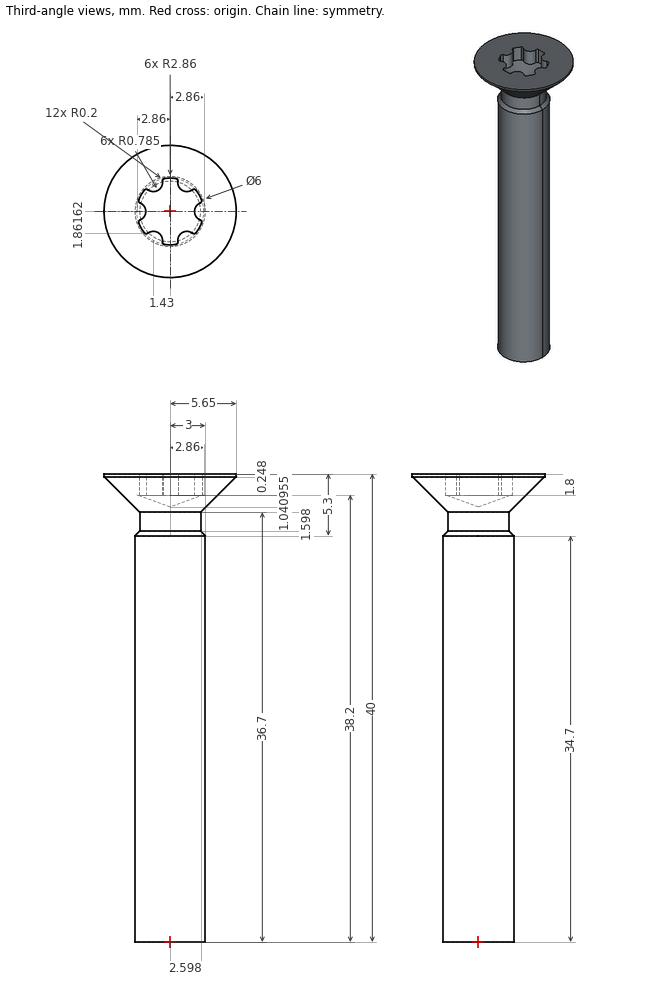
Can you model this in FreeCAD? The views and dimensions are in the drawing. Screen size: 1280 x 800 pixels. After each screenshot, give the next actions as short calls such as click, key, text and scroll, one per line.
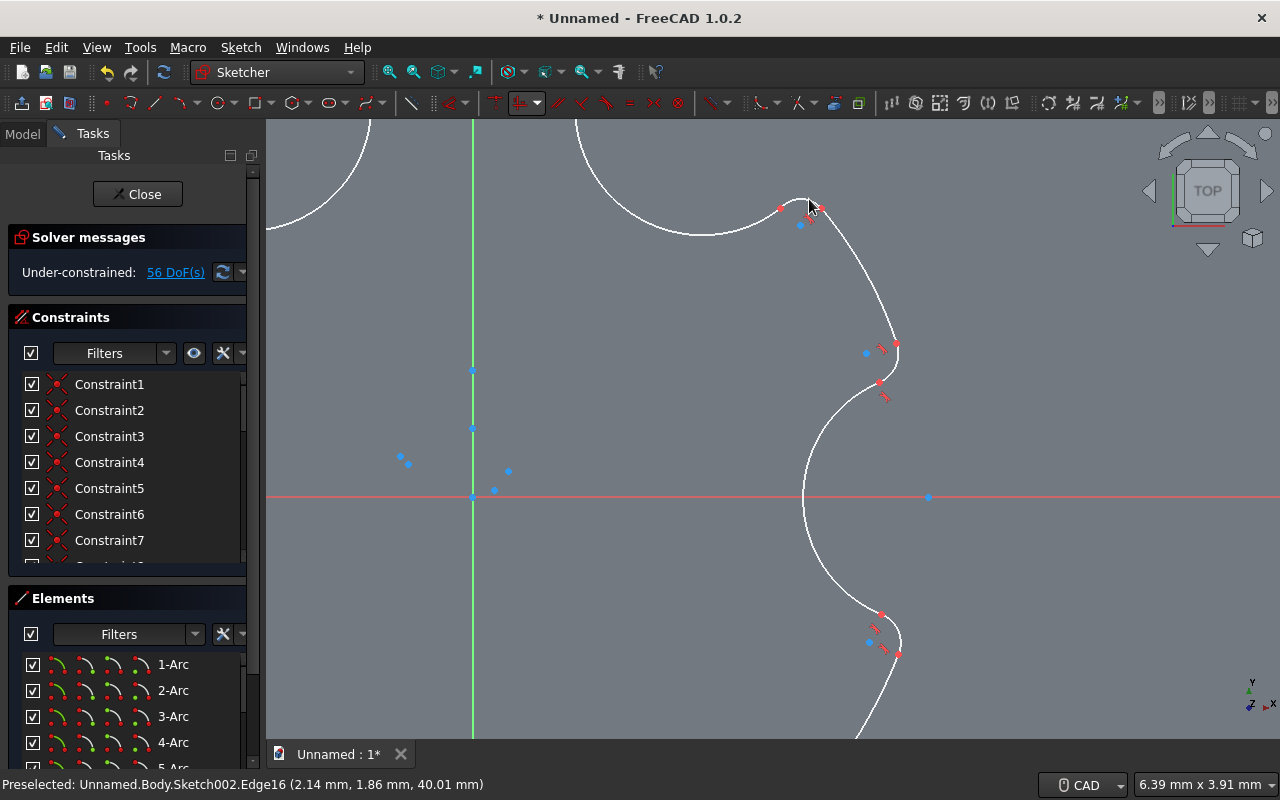
click(810, 201)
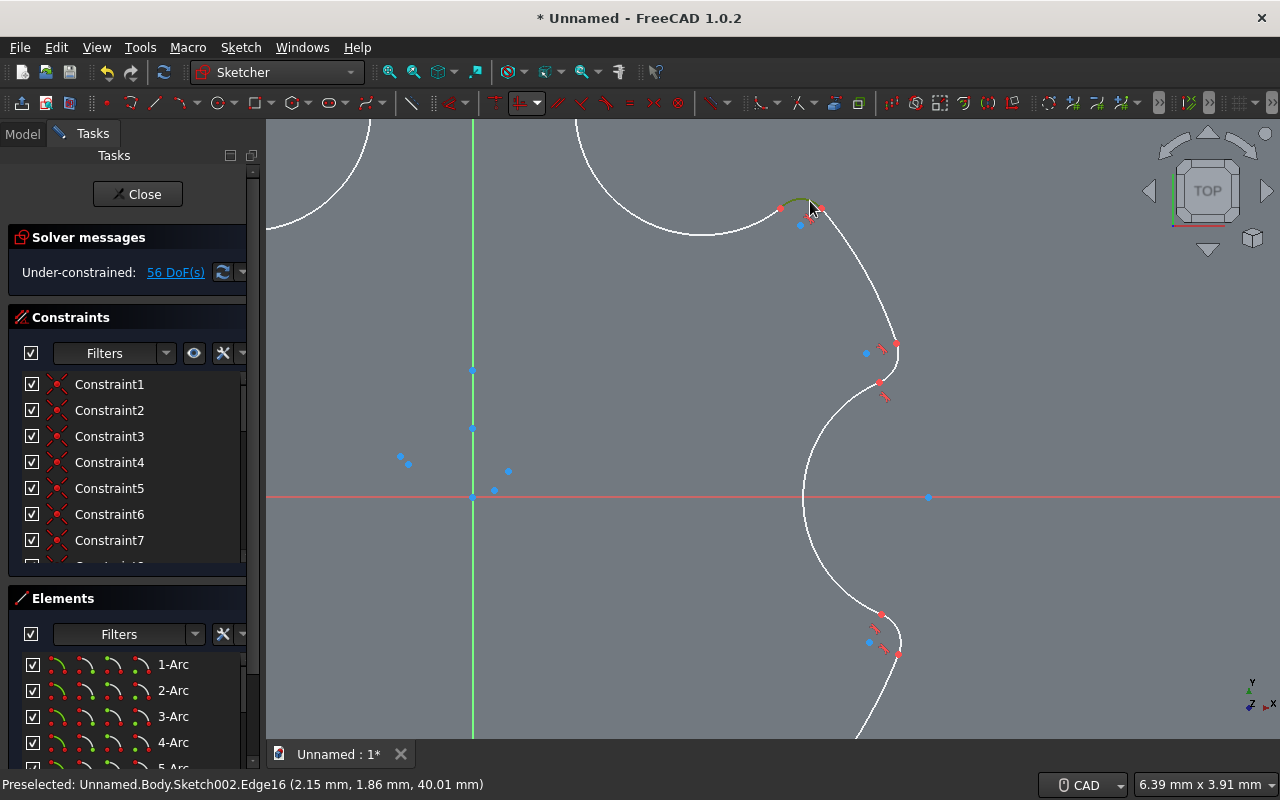
click(594, 175)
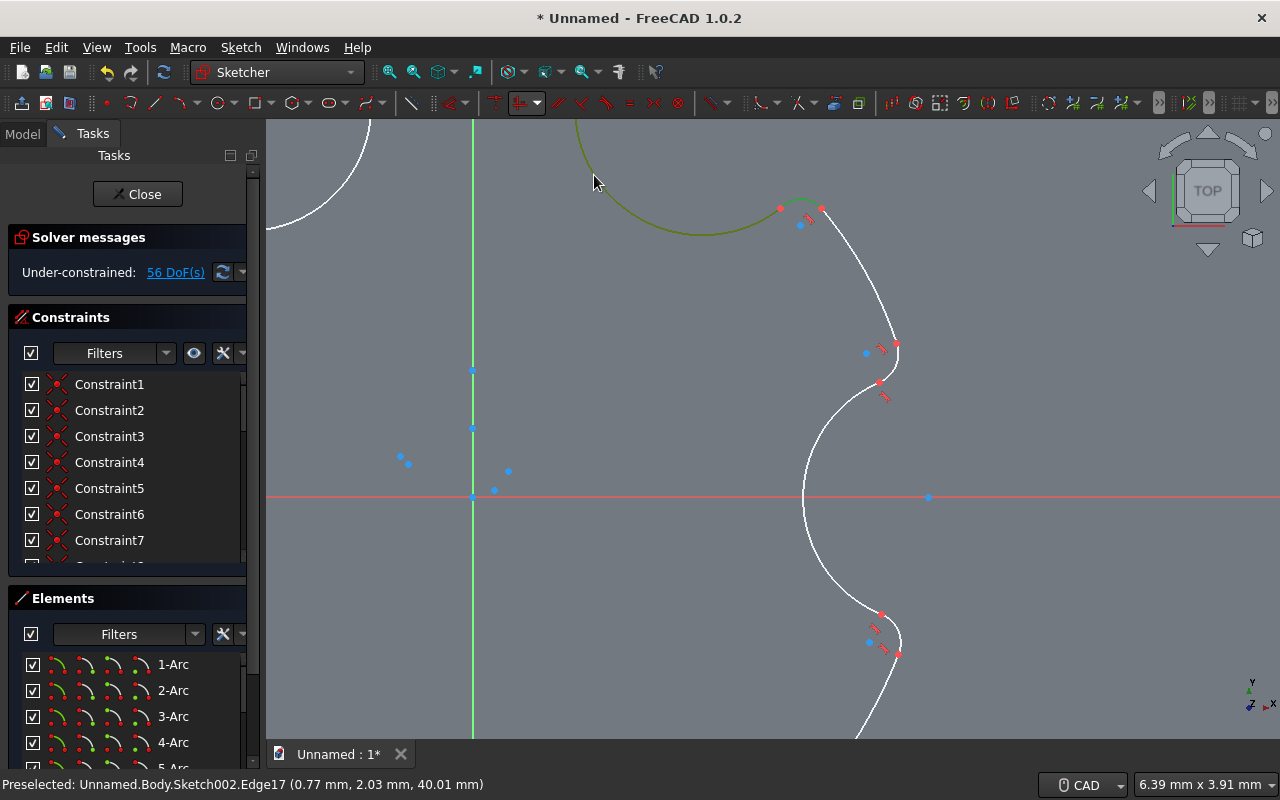
key(t)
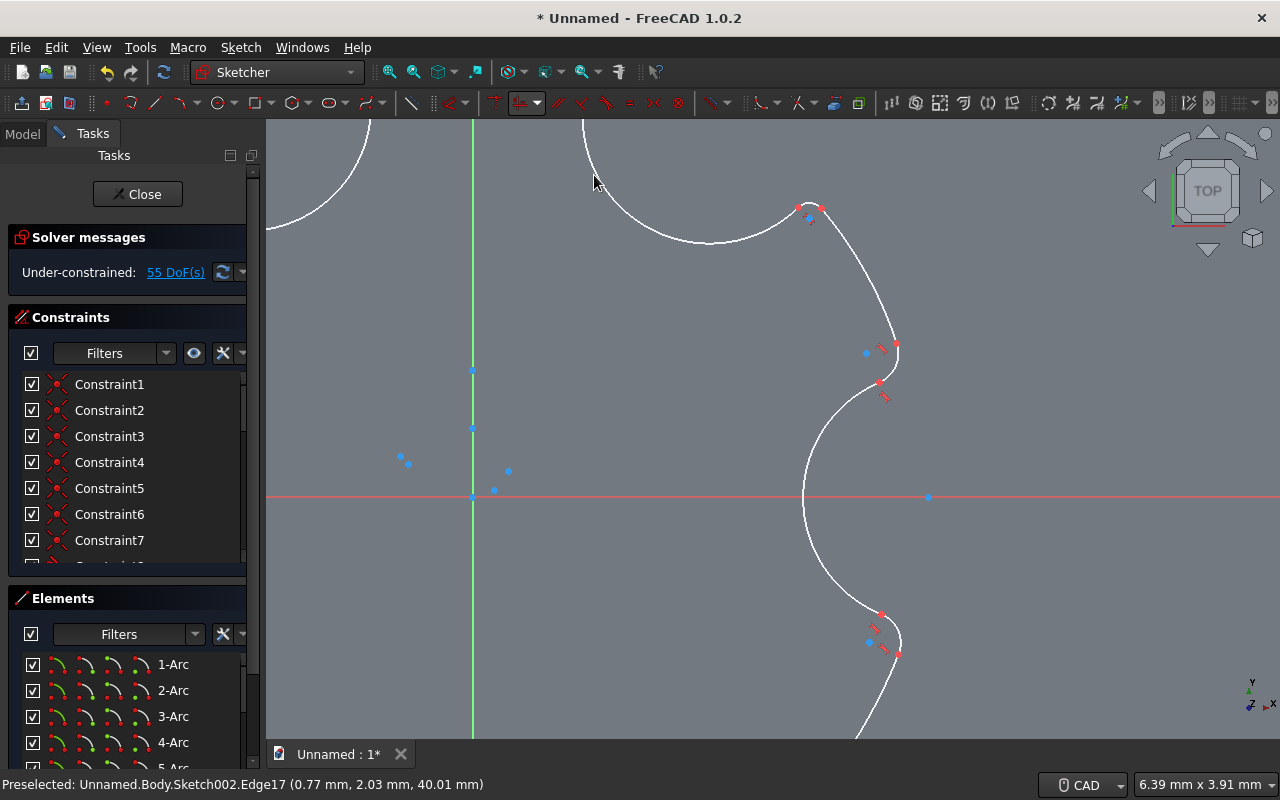
click(604, 187)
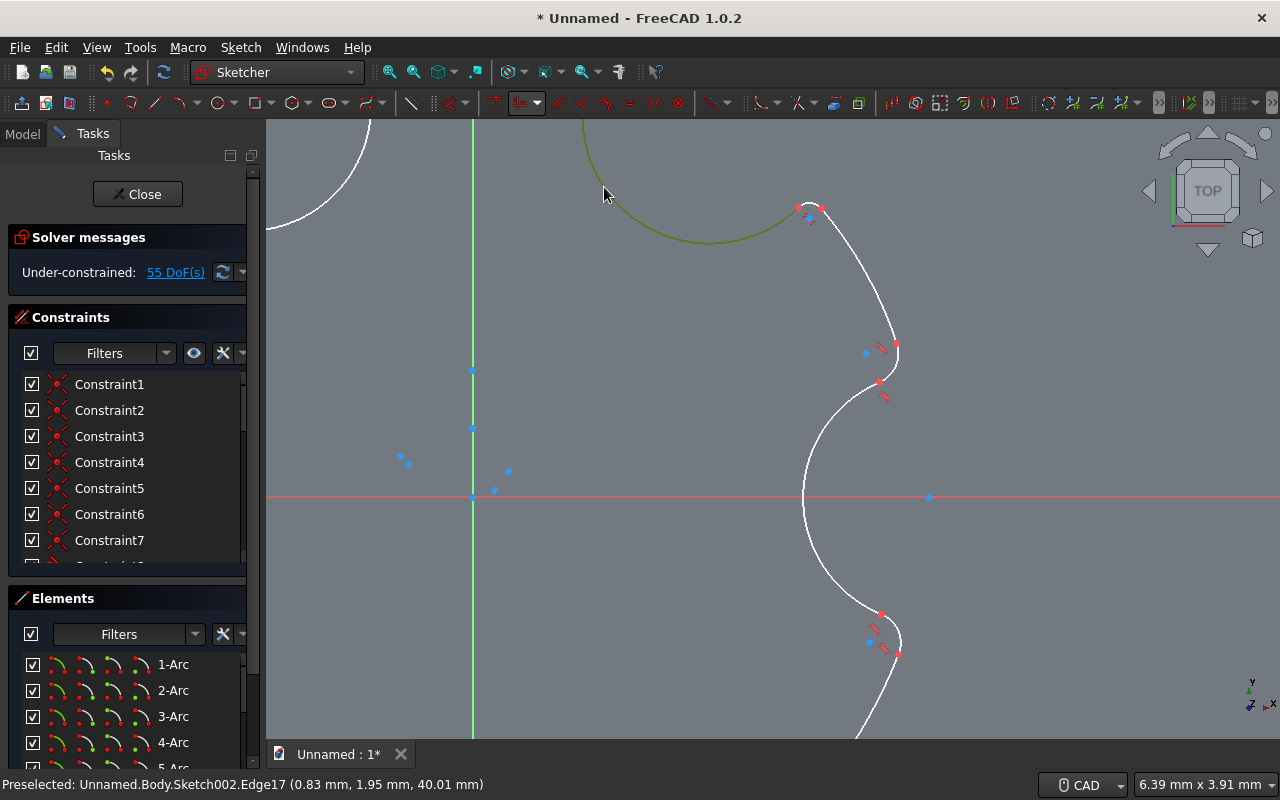
scroll(894, 373, down, 4)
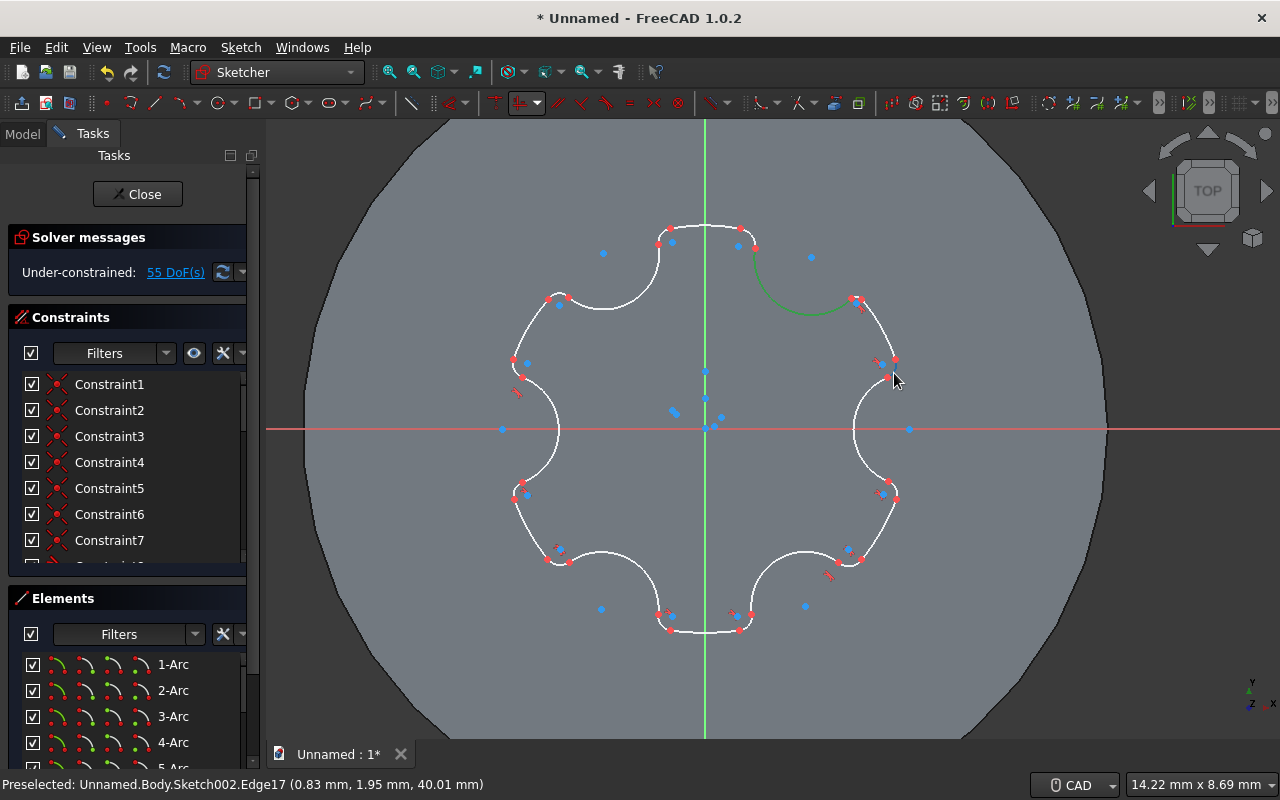
scroll(754, 241, up, 3)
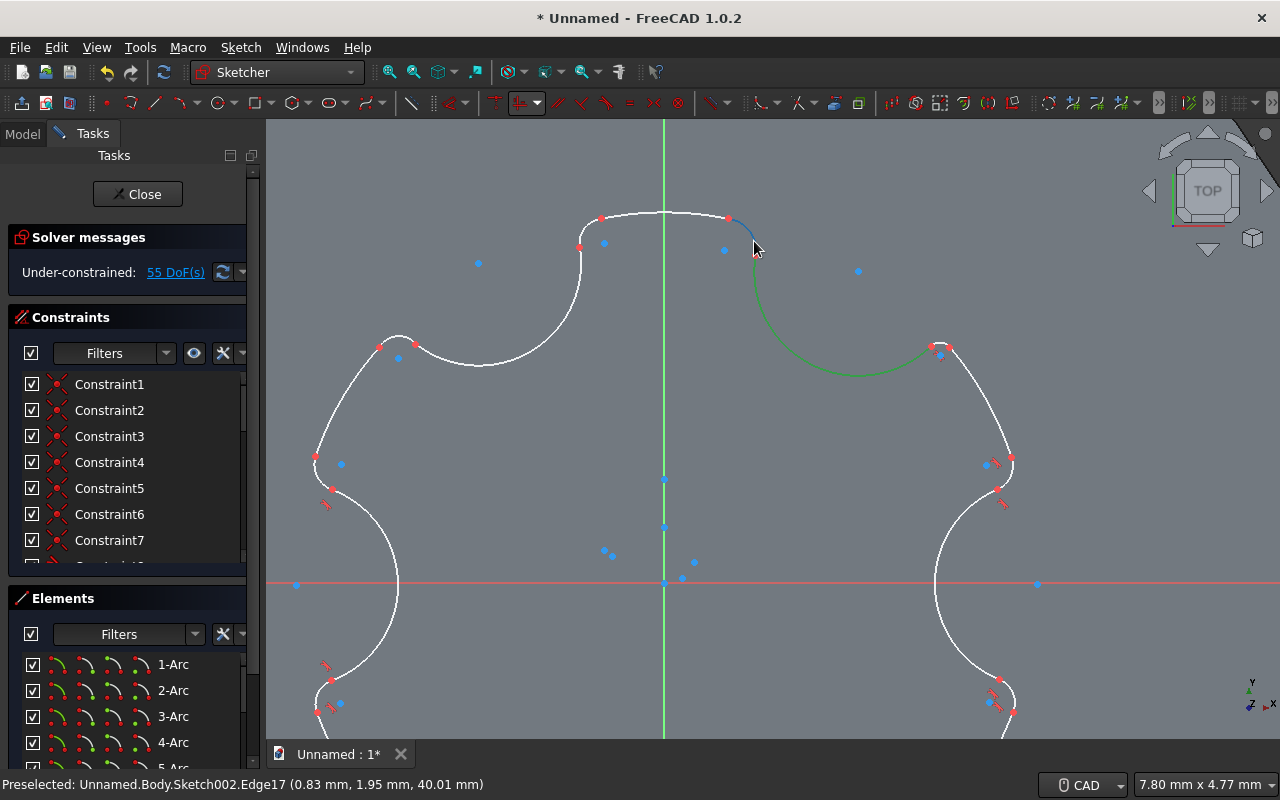
click(754, 240)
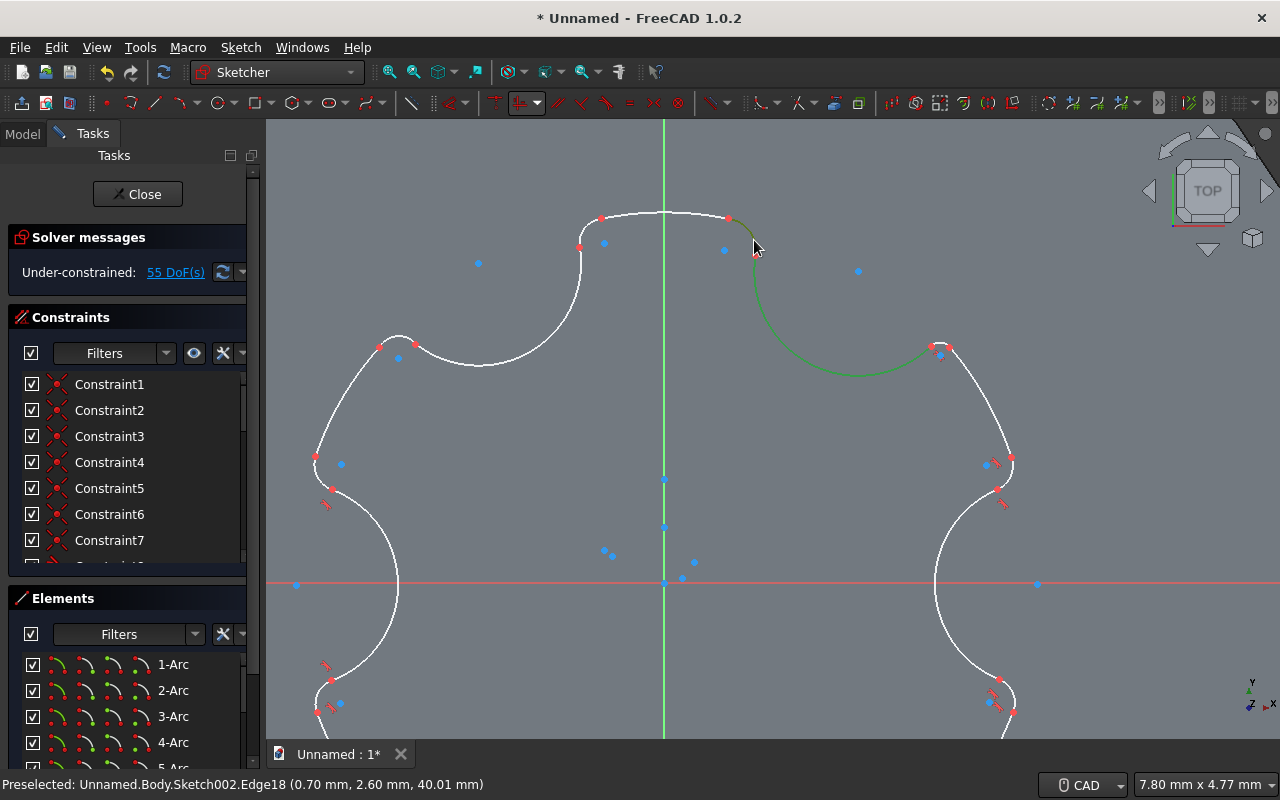
click(606, 104)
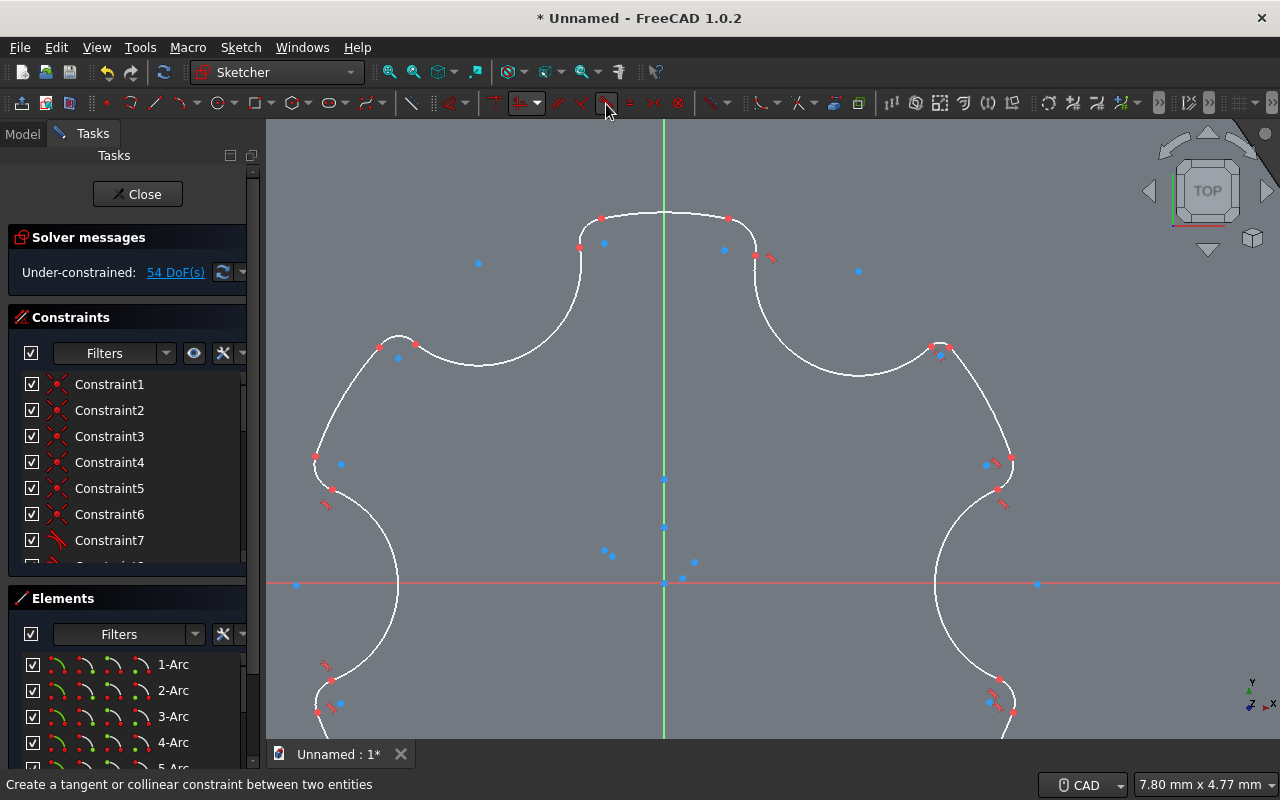
click(755, 240)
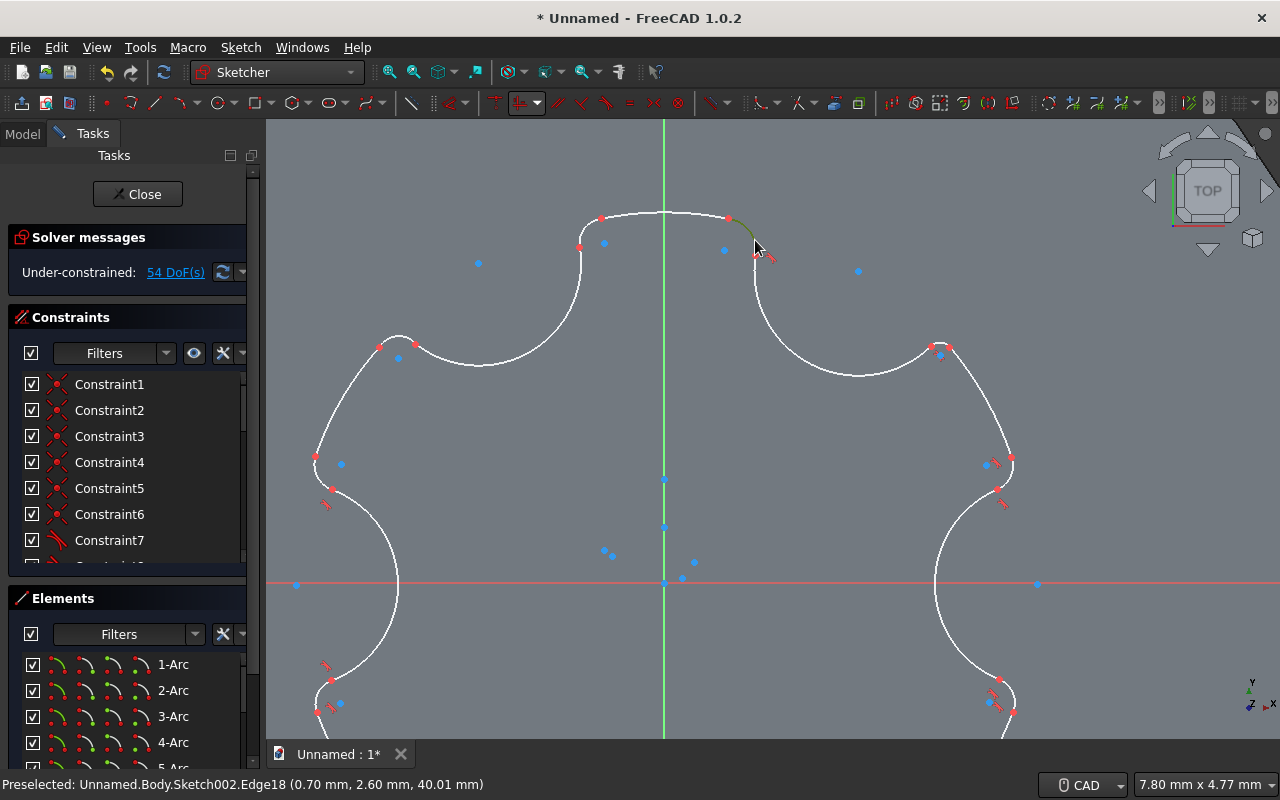
click(690, 213)